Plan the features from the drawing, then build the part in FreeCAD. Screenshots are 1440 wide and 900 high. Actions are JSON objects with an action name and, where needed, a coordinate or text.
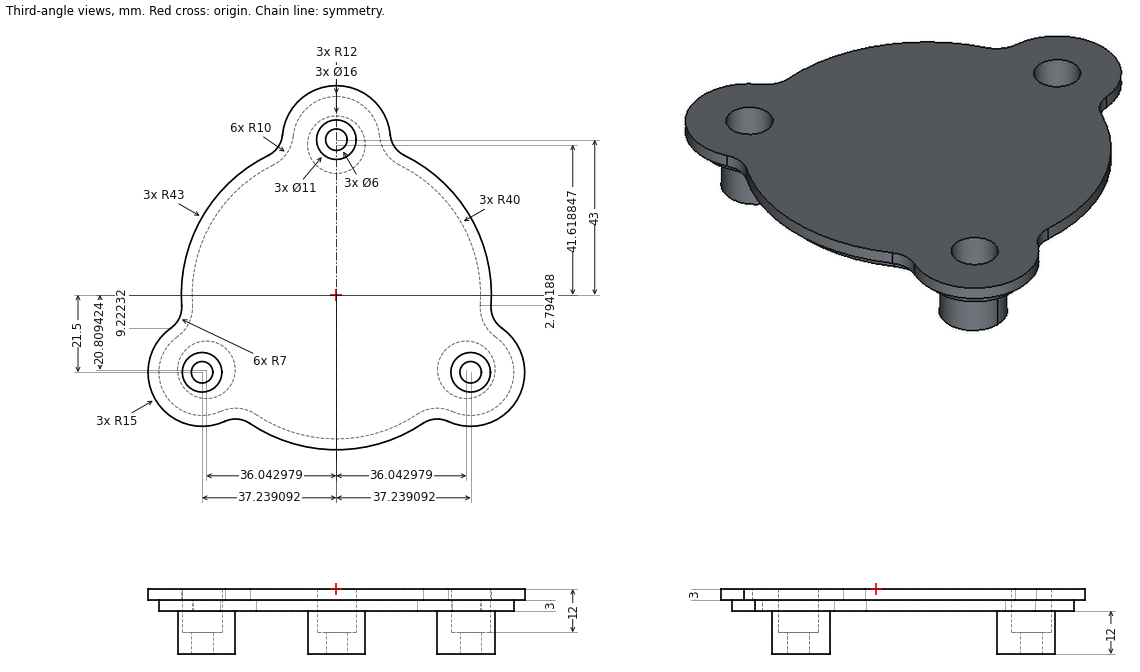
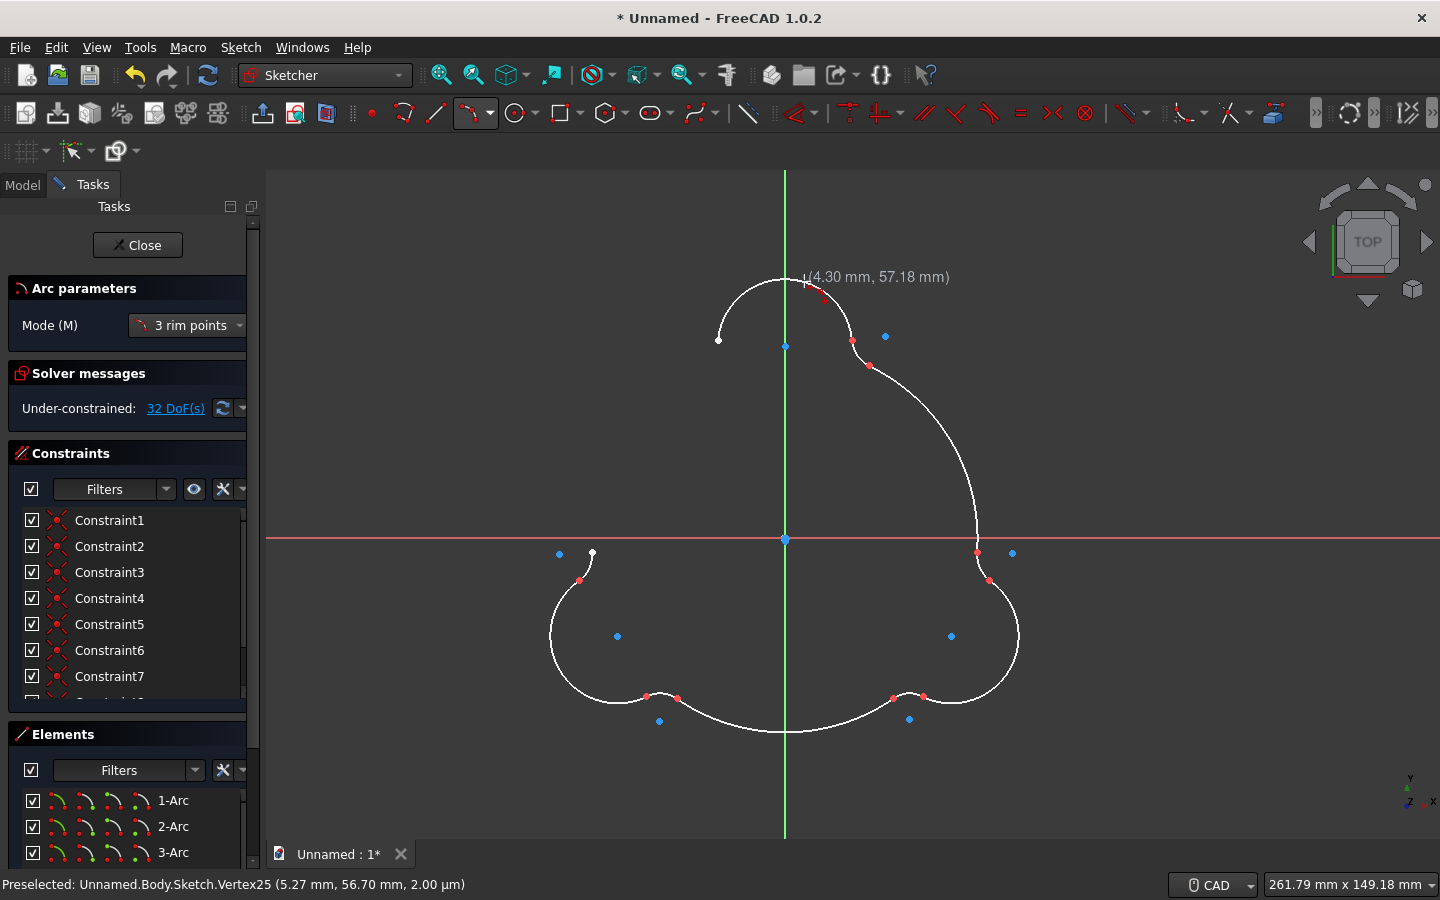
{"action": "left_click", "coordinate": [718, 341]}
{"action": "left_click", "coordinate": [700, 365]}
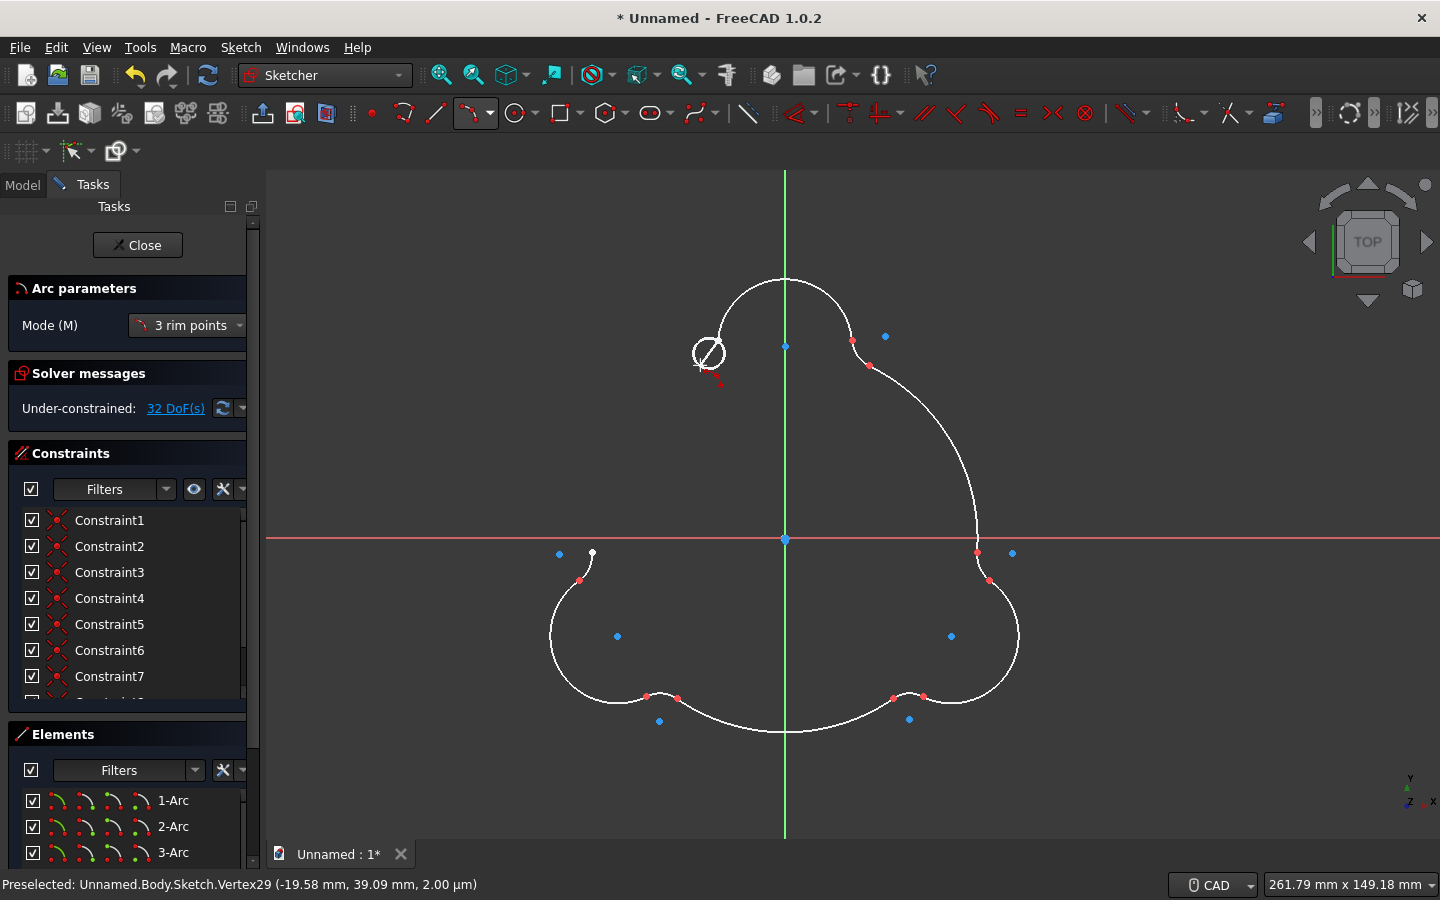
{"action": "scroll", "coordinate": [712, 355], "scroll_direction": "up", "scroll_amount": 7}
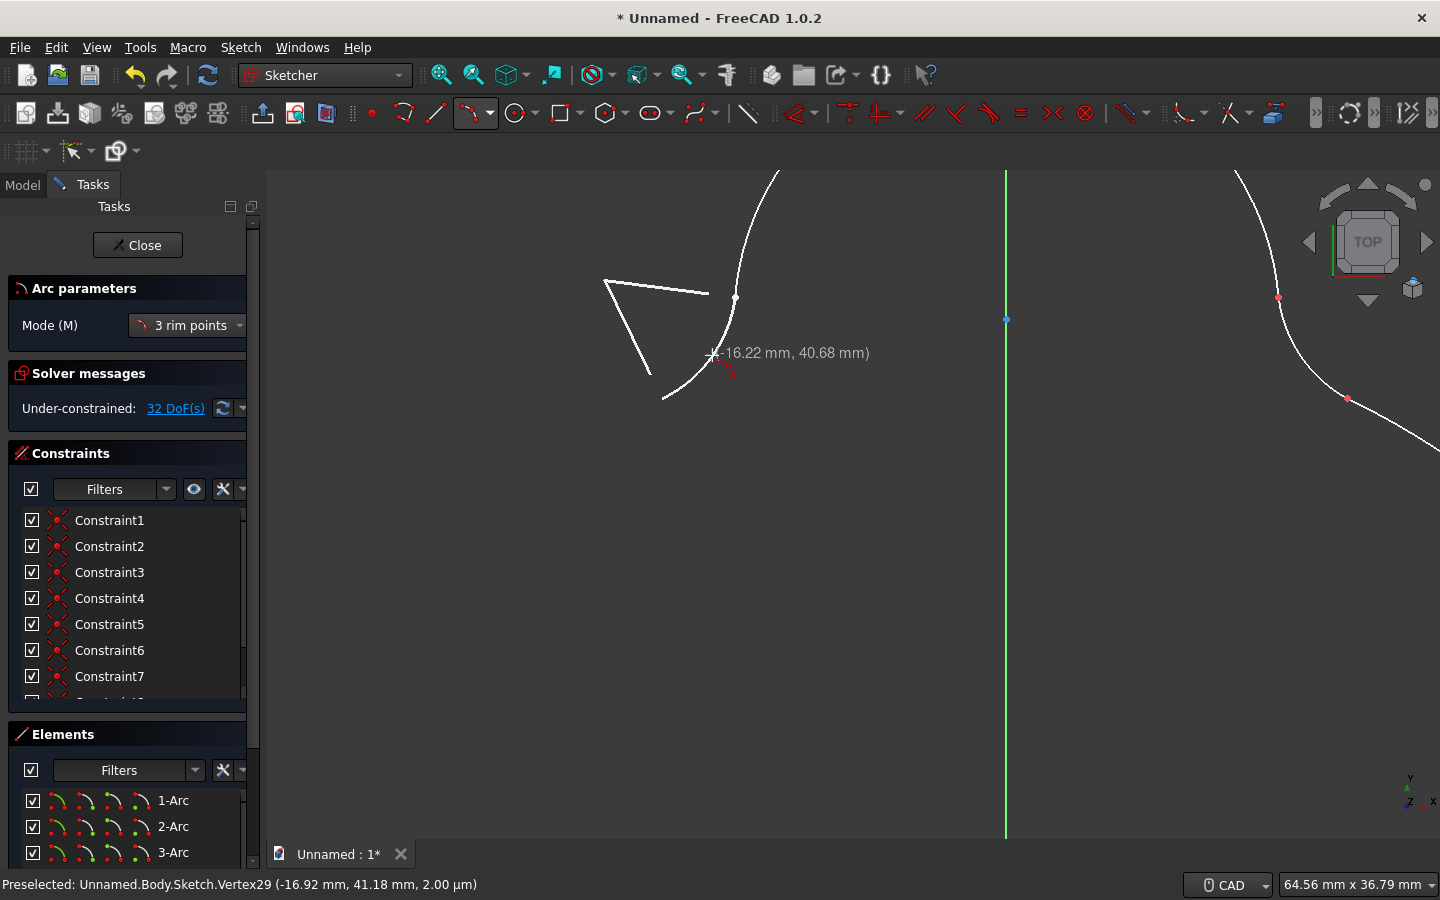
{"action": "left_click", "coordinate": [712, 353]}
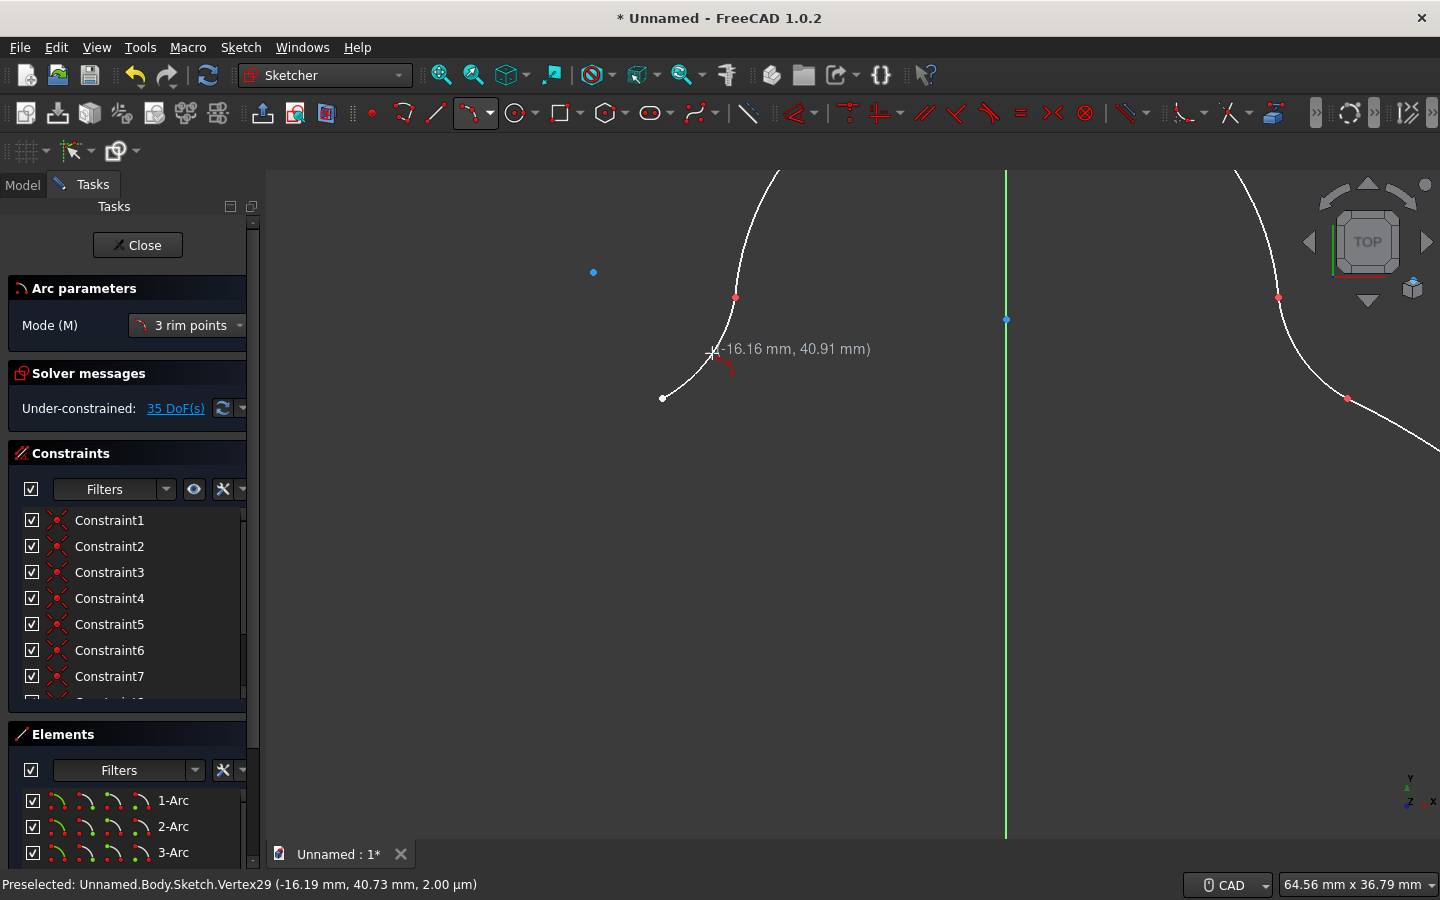
{"action": "scroll", "coordinate": [712, 355], "scroll_direction": "down", "scroll_amount": 7}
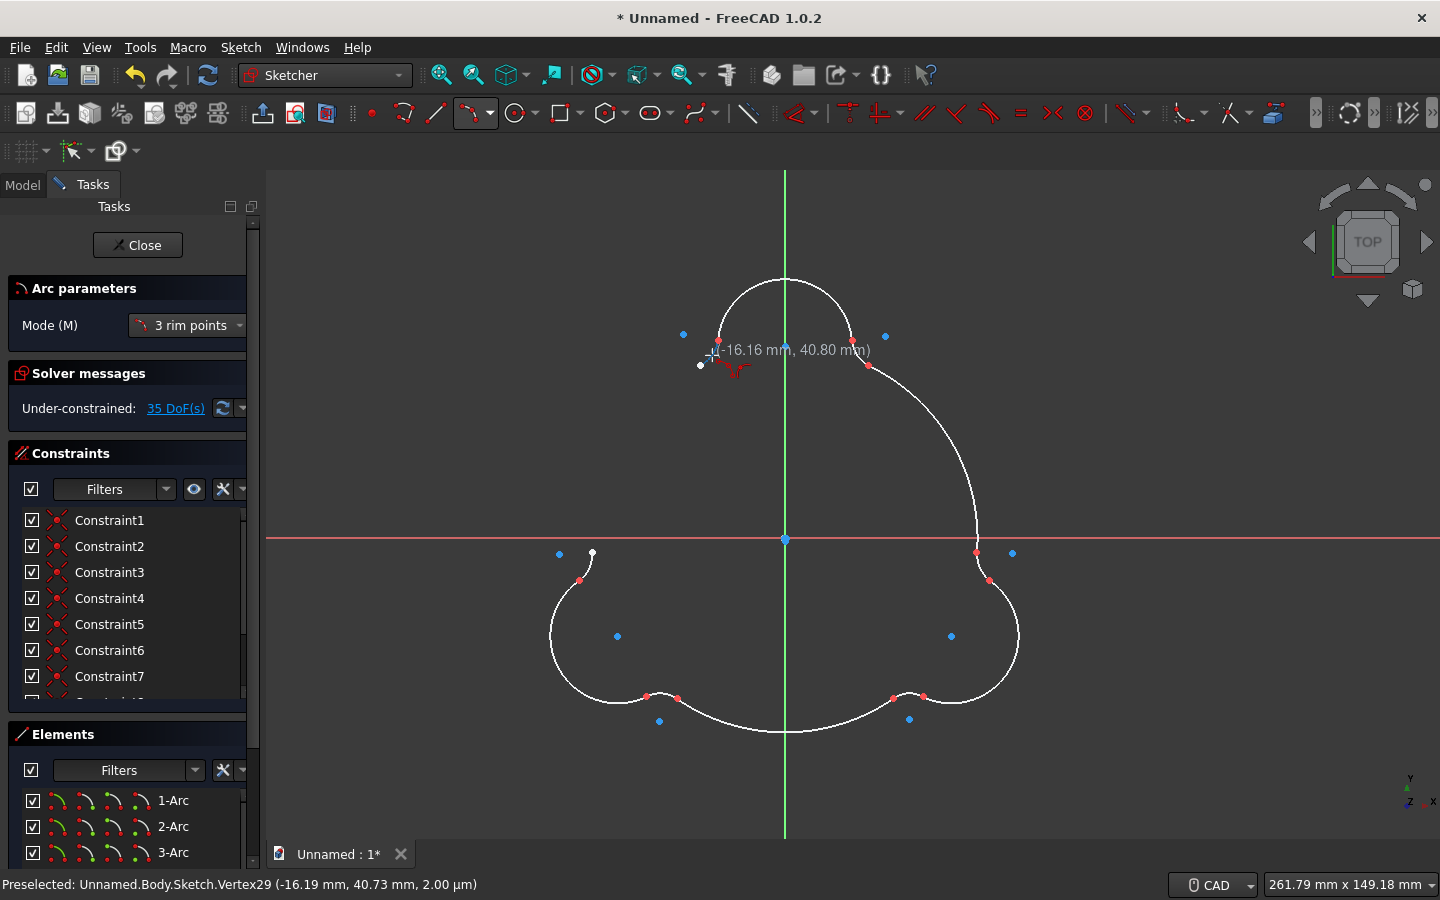
{"action": "left_click", "coordinate": [700, 366]}
{"action": "left_click", "coordinate": [592, 553]}
{"action": "left_click", "coordinate": [618, 442]}
{"action": "key", "text": "Escape"}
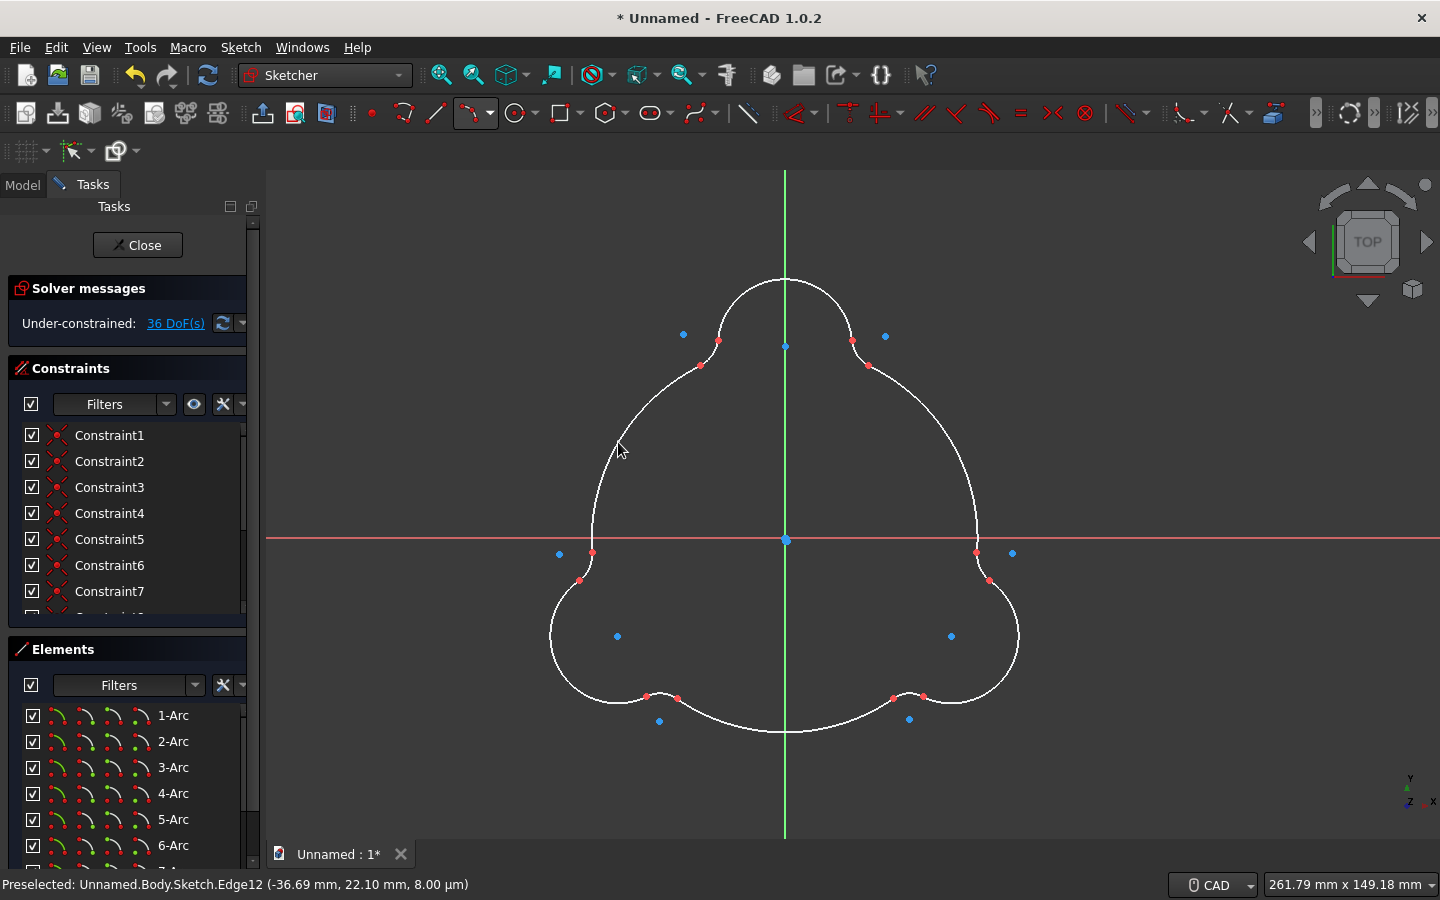
{"action": "scroll", "coordinate": [586, 574], "scroll_direction": "up", "scroll_amount": 2}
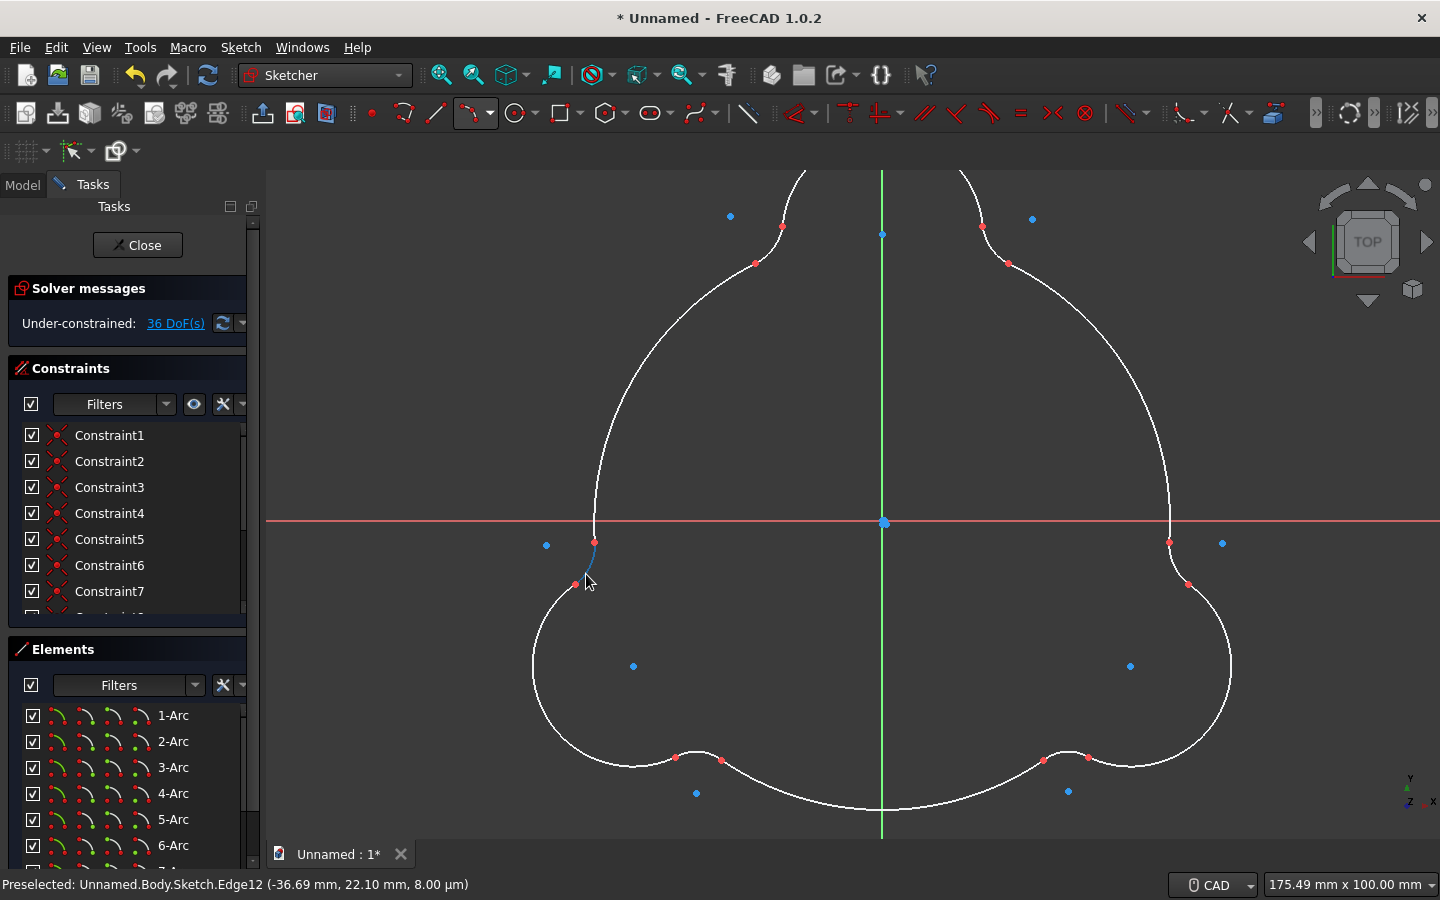
{"action": "left_click", "coordinate": [586, 574]}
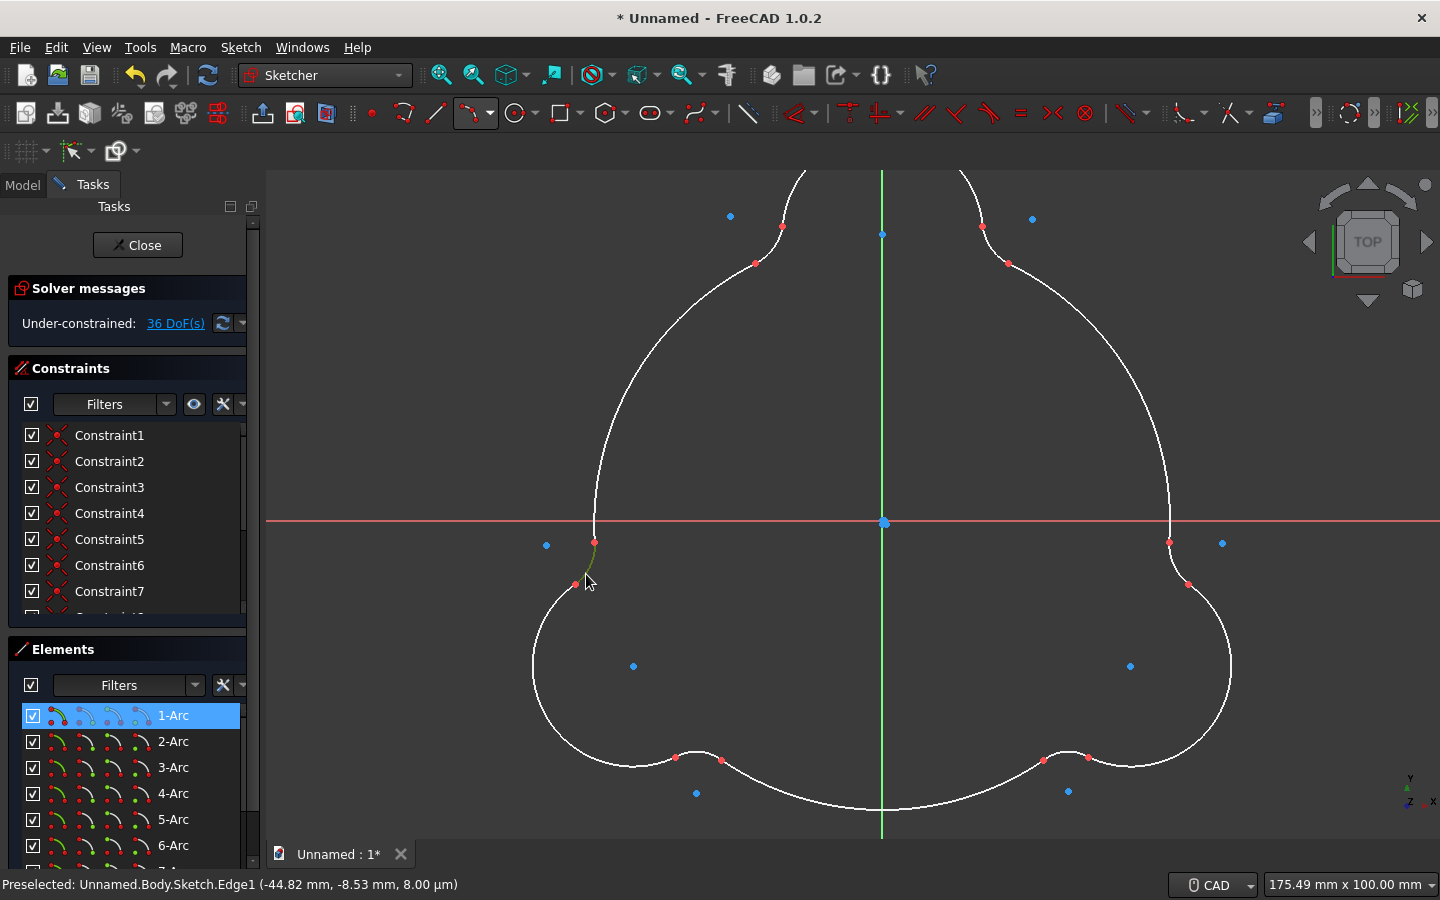
{"action": "left_click", "coordinate": [533, 659]}